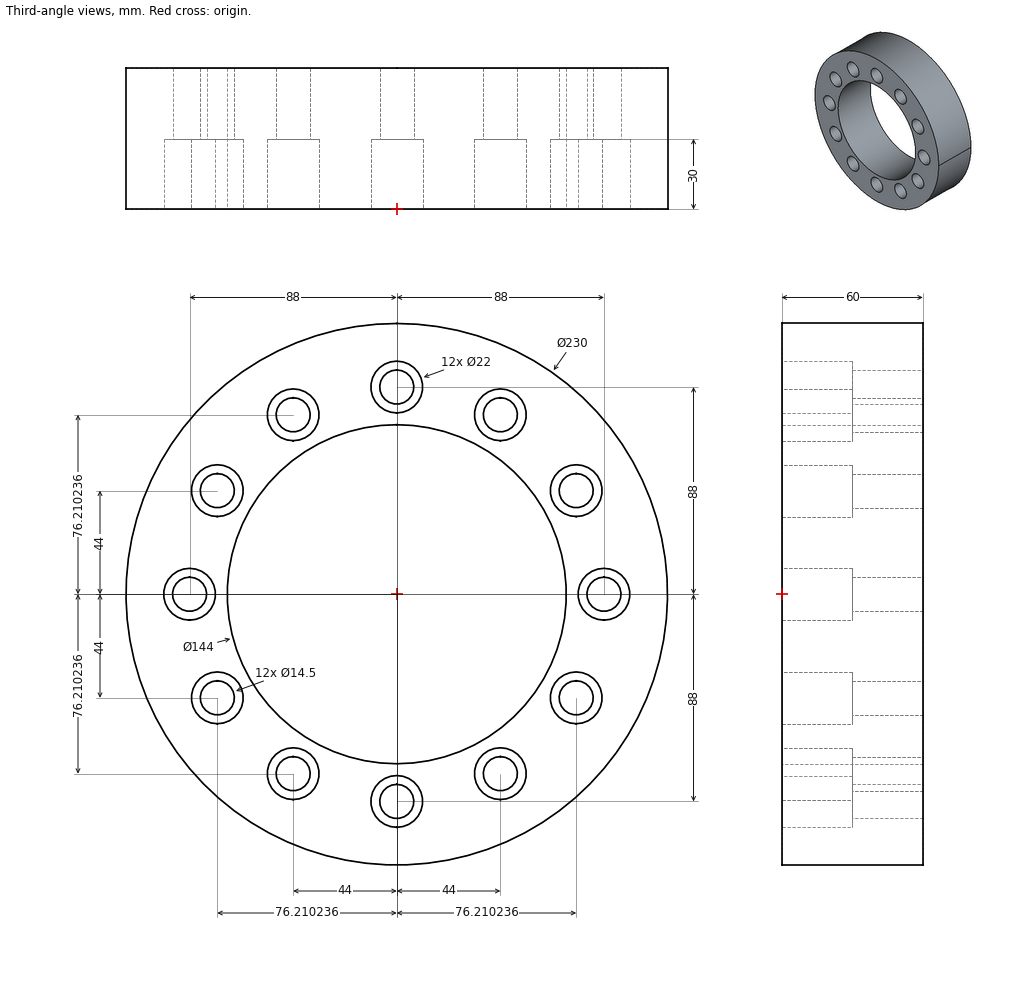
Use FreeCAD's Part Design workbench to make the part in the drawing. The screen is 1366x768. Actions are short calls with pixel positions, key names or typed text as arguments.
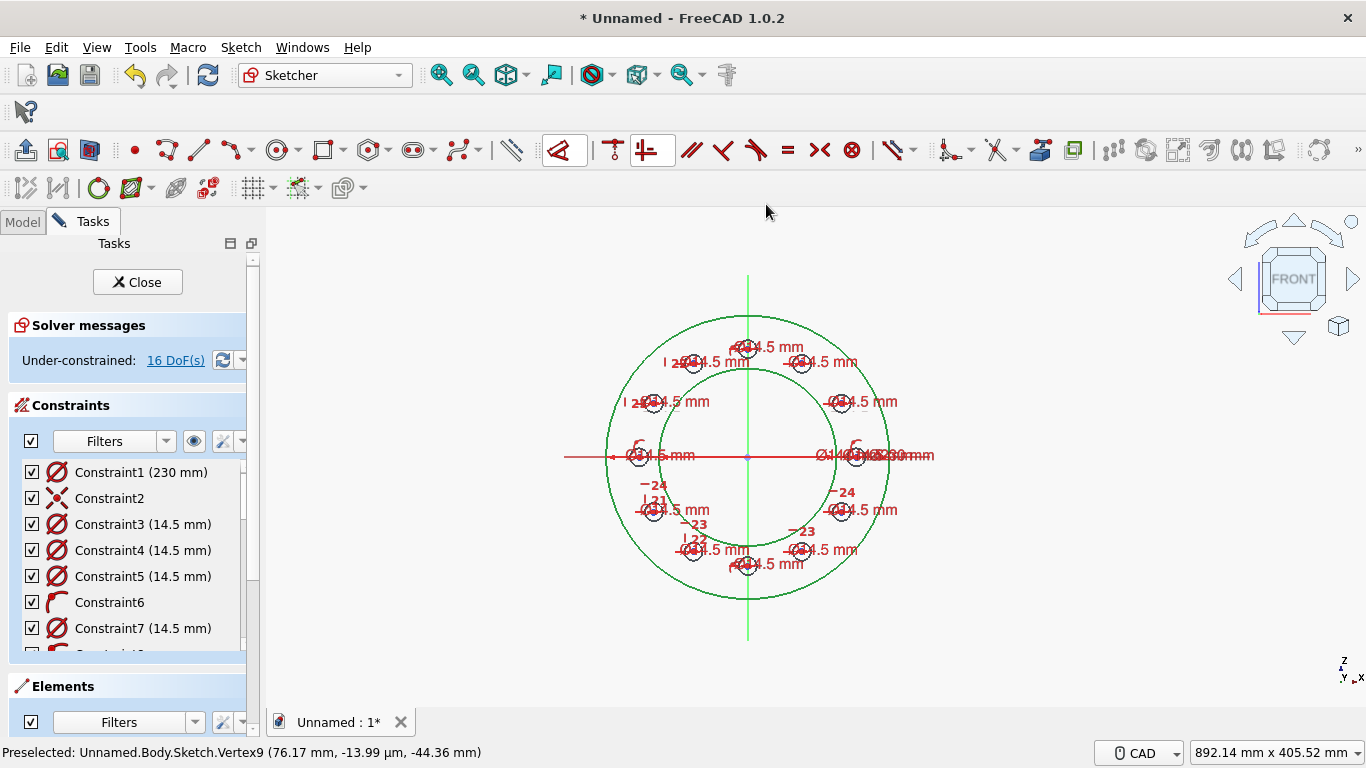
click(694, 364)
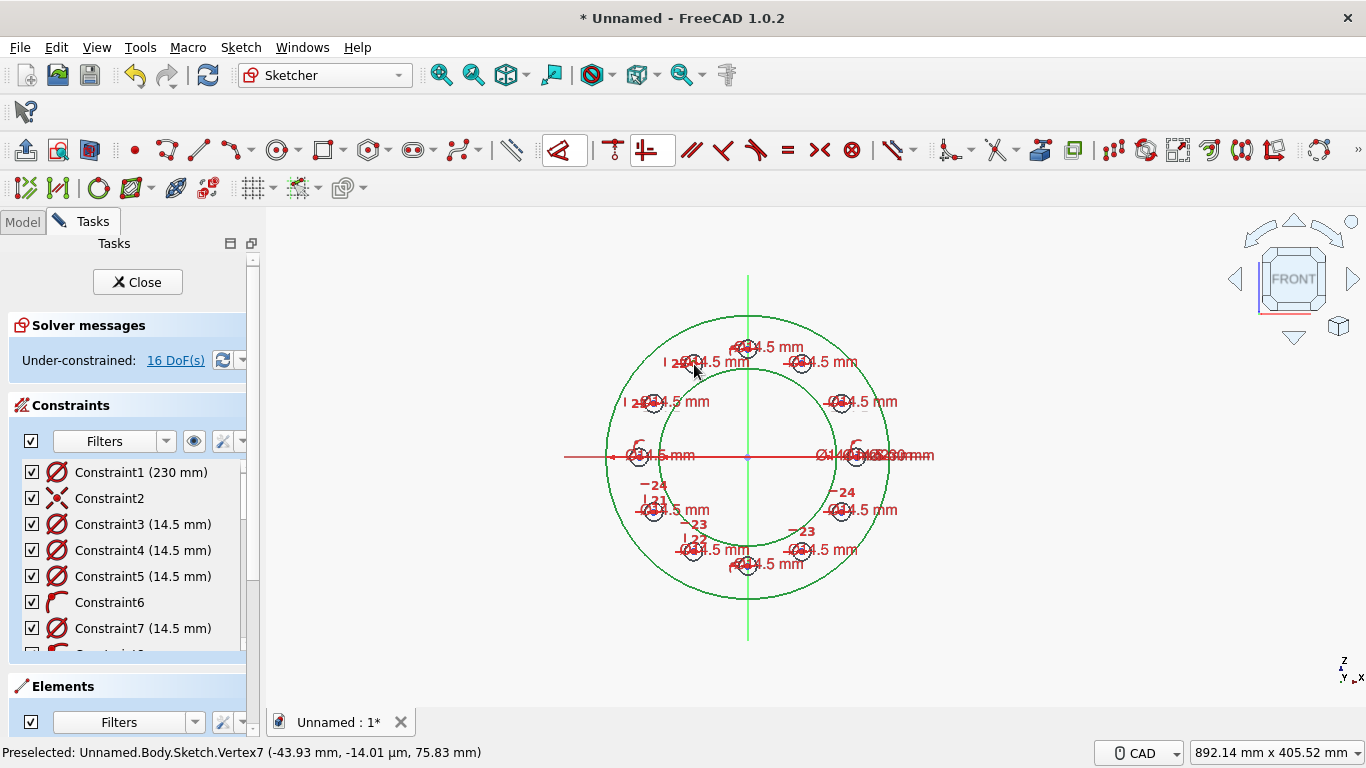
click(802, 364)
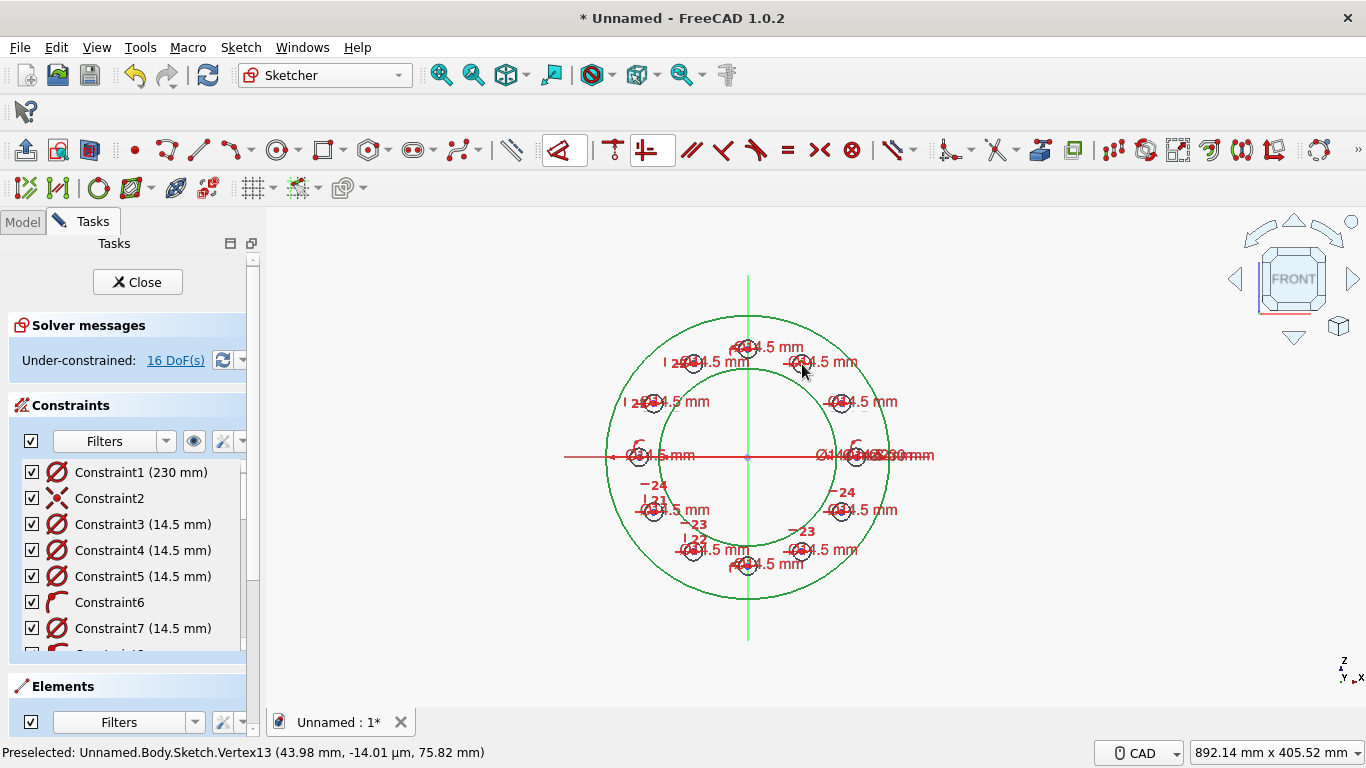
click(670, 150)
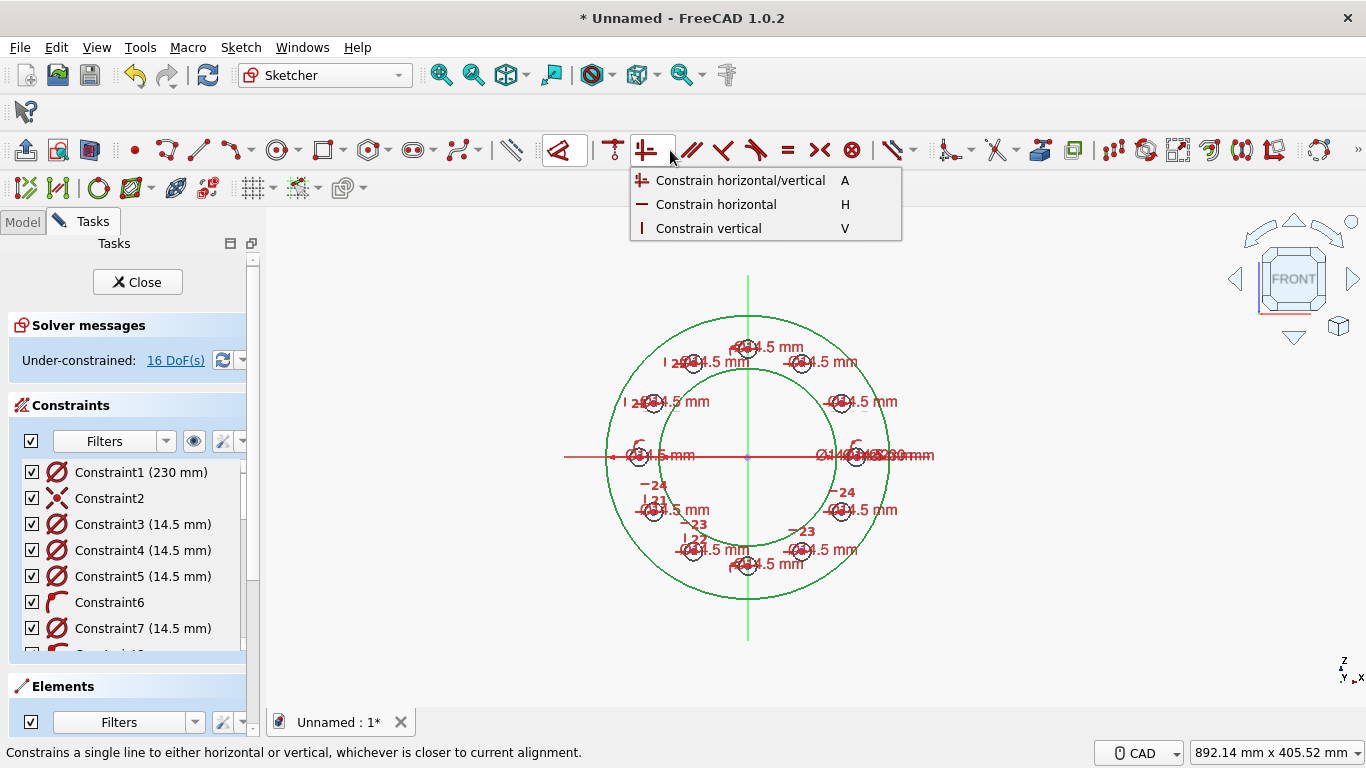
click(766, 204)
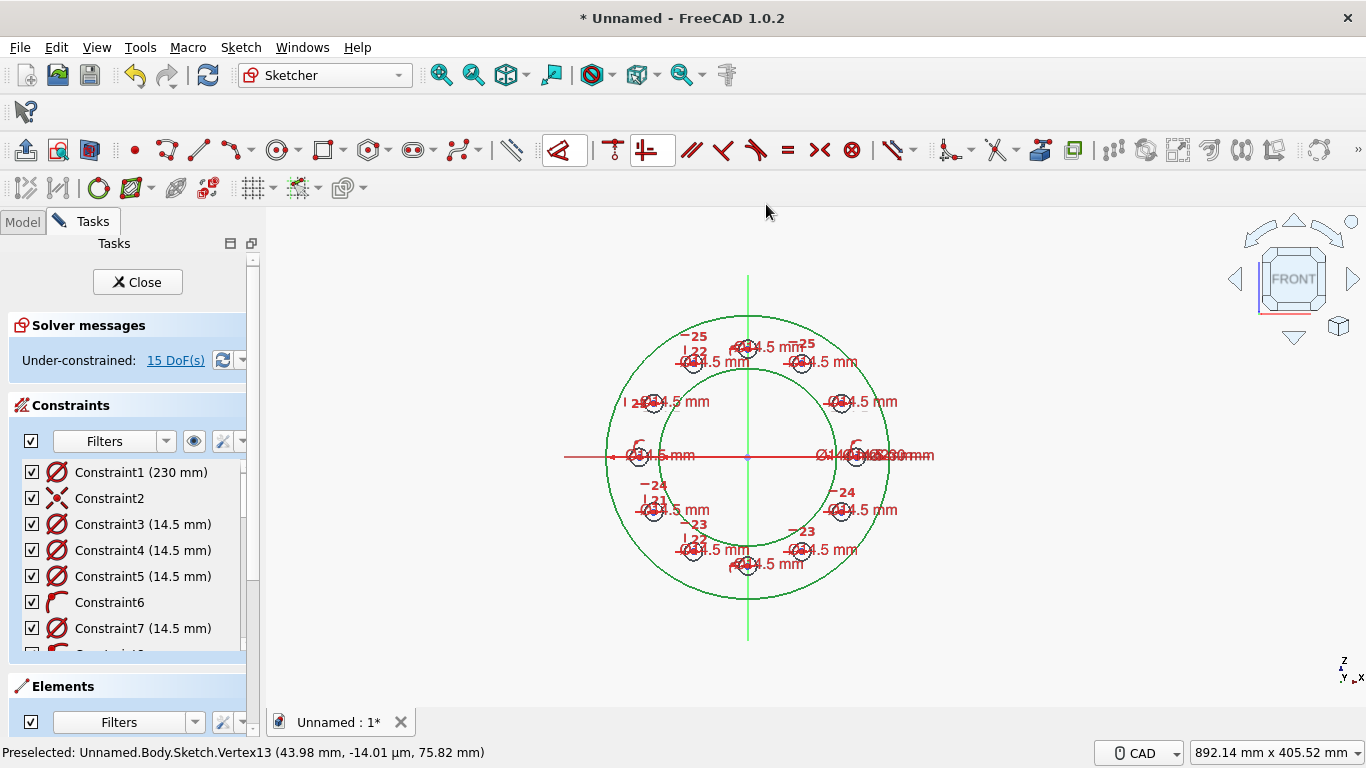
click(842, 512)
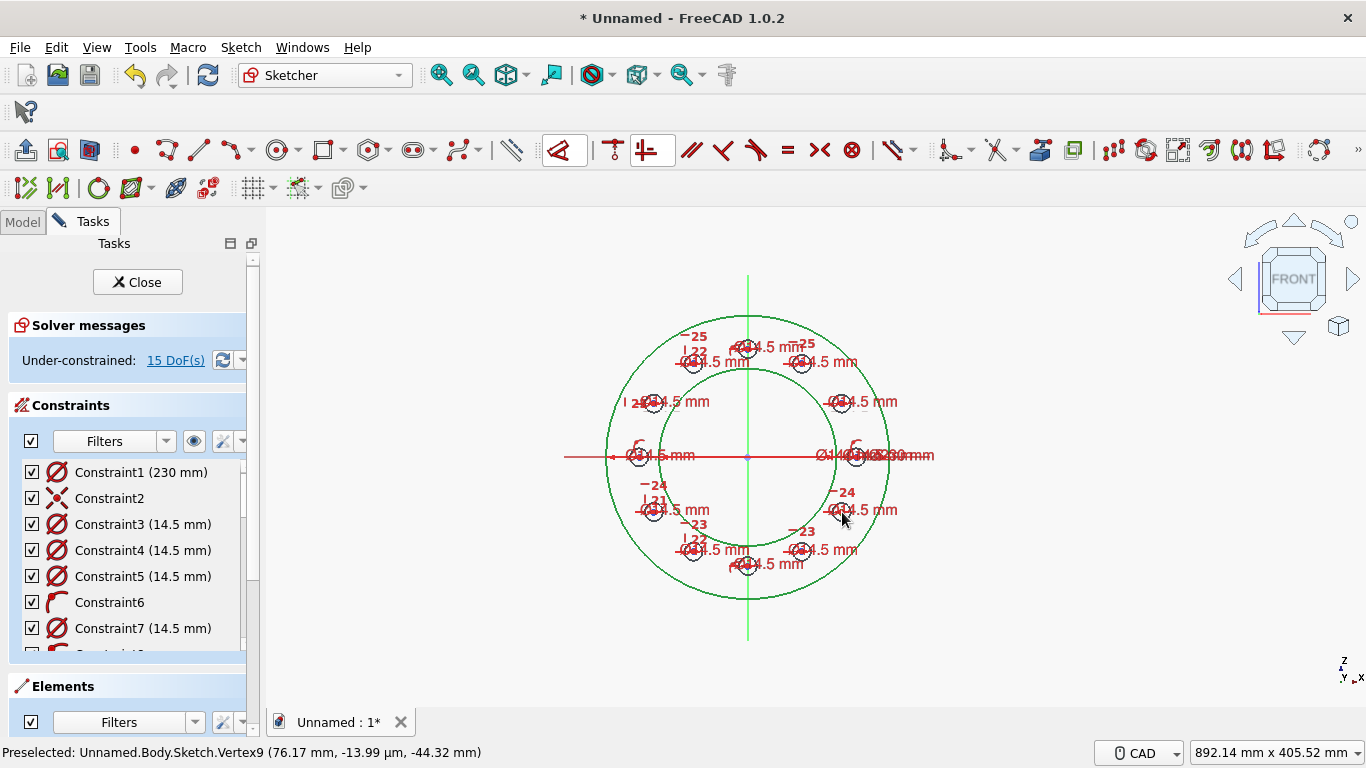
click(842, 404)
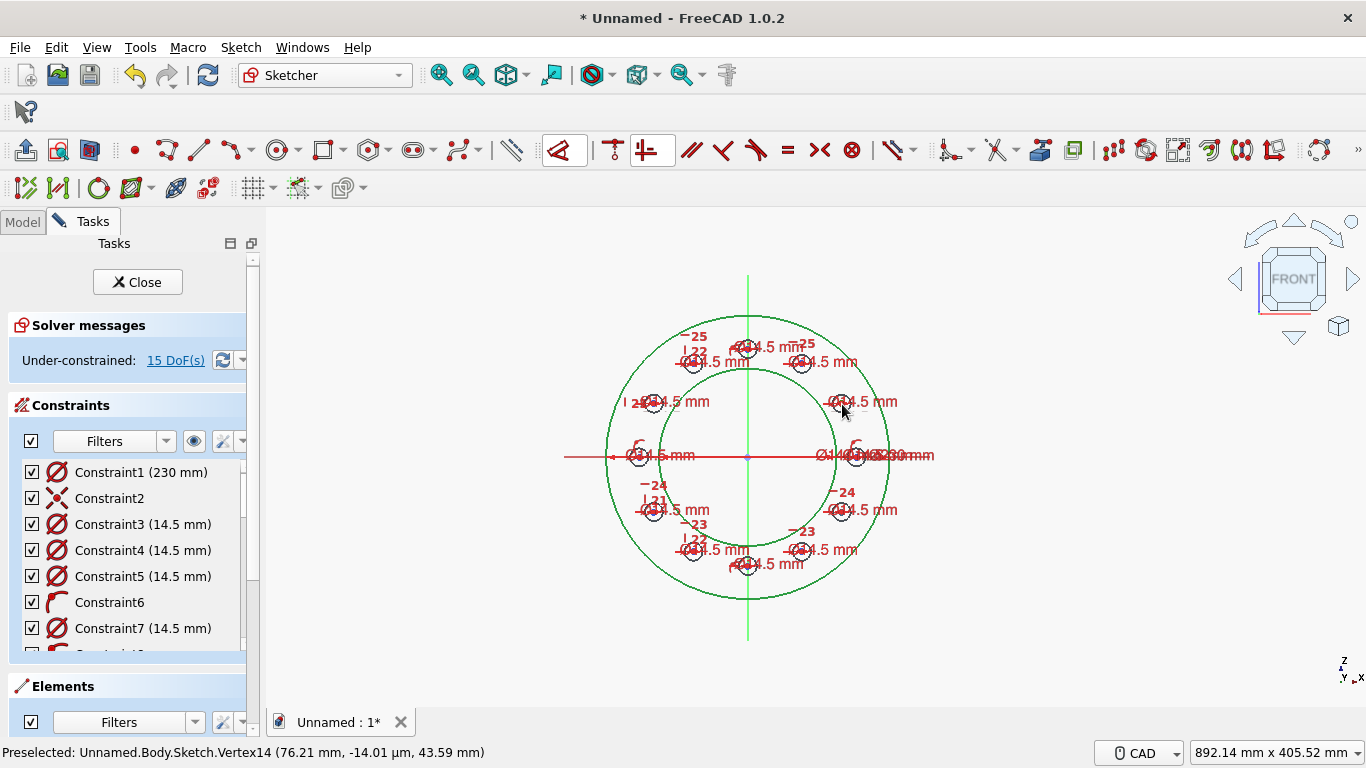
key(v)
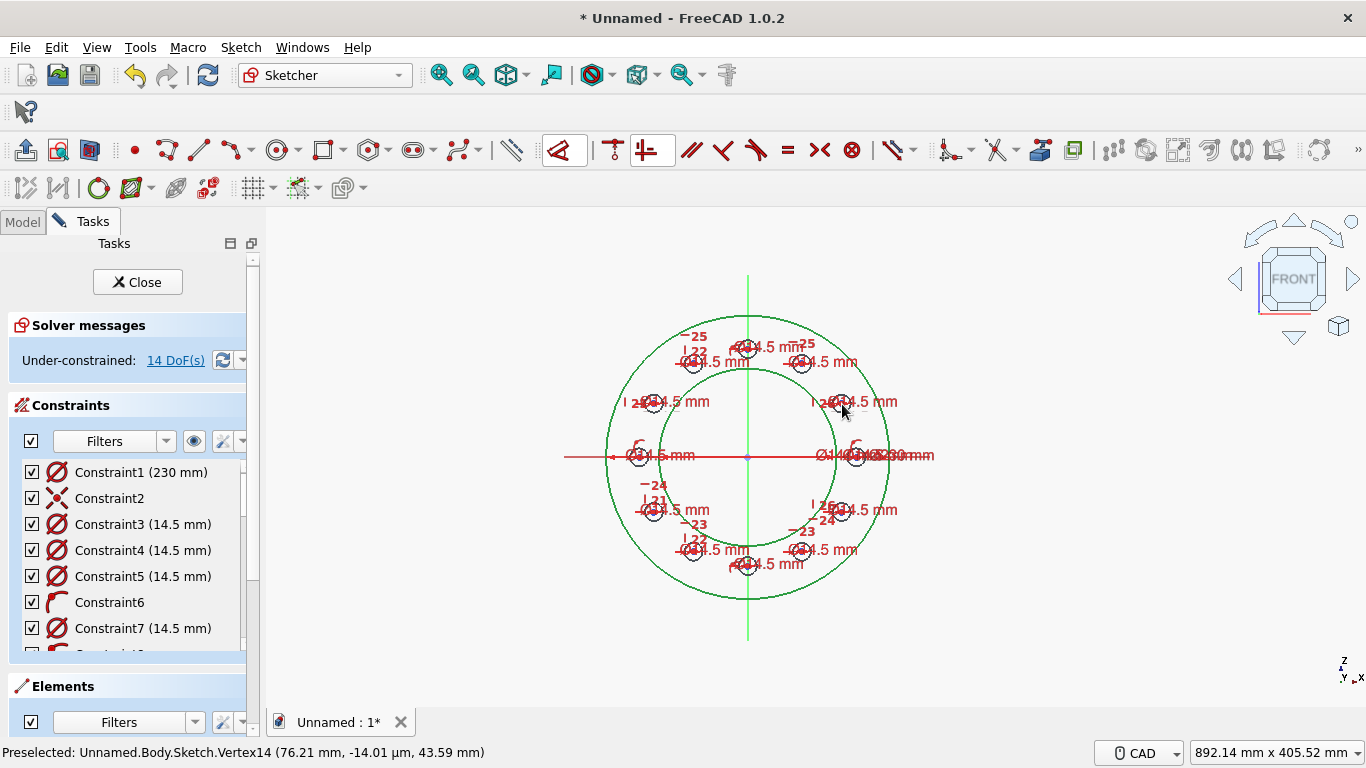
click(558, 150)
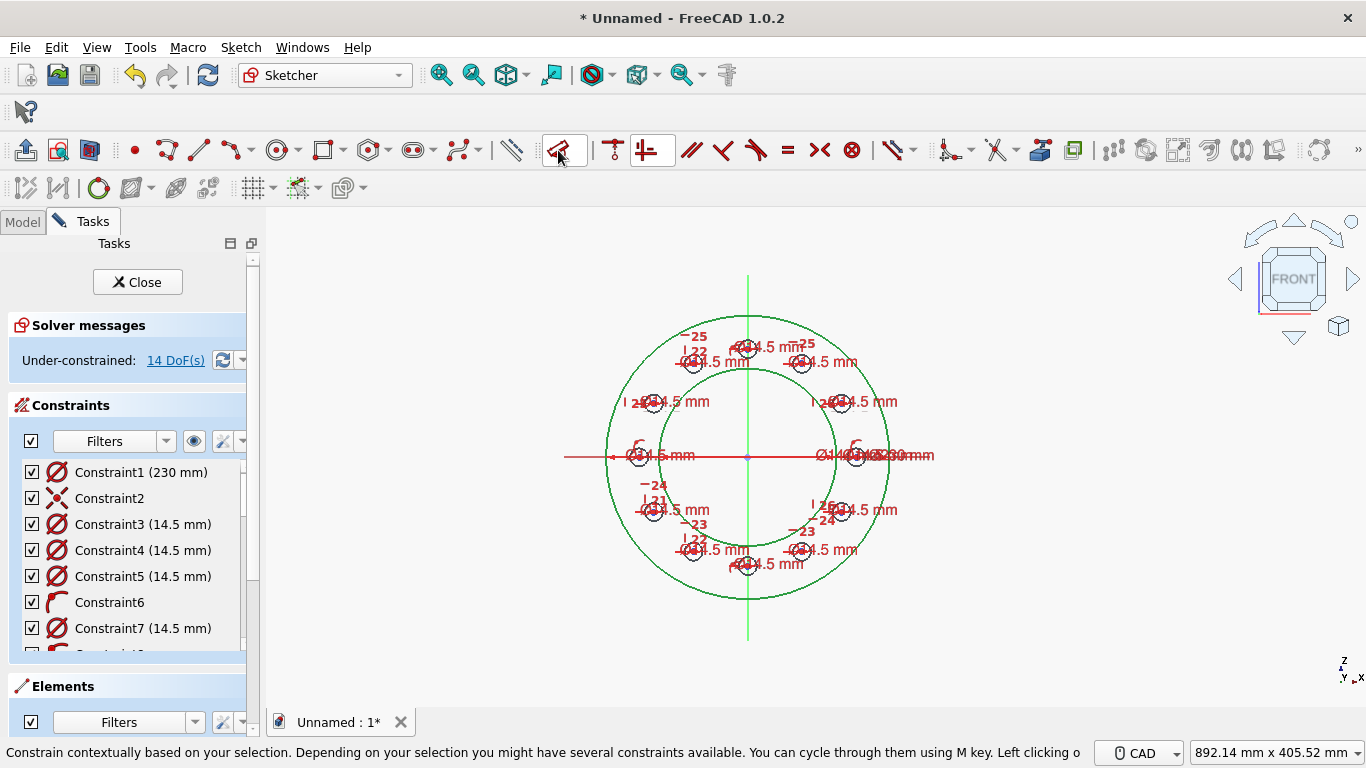
click(654, 512)
click(620, 472)